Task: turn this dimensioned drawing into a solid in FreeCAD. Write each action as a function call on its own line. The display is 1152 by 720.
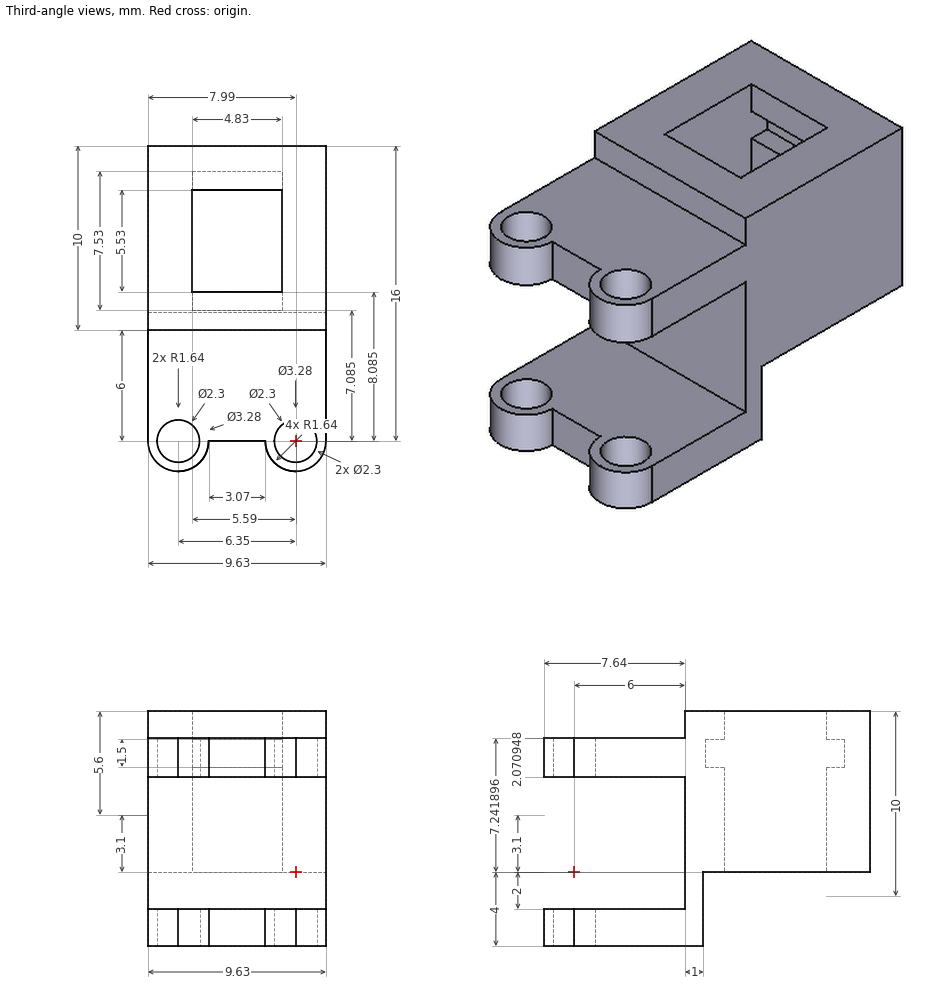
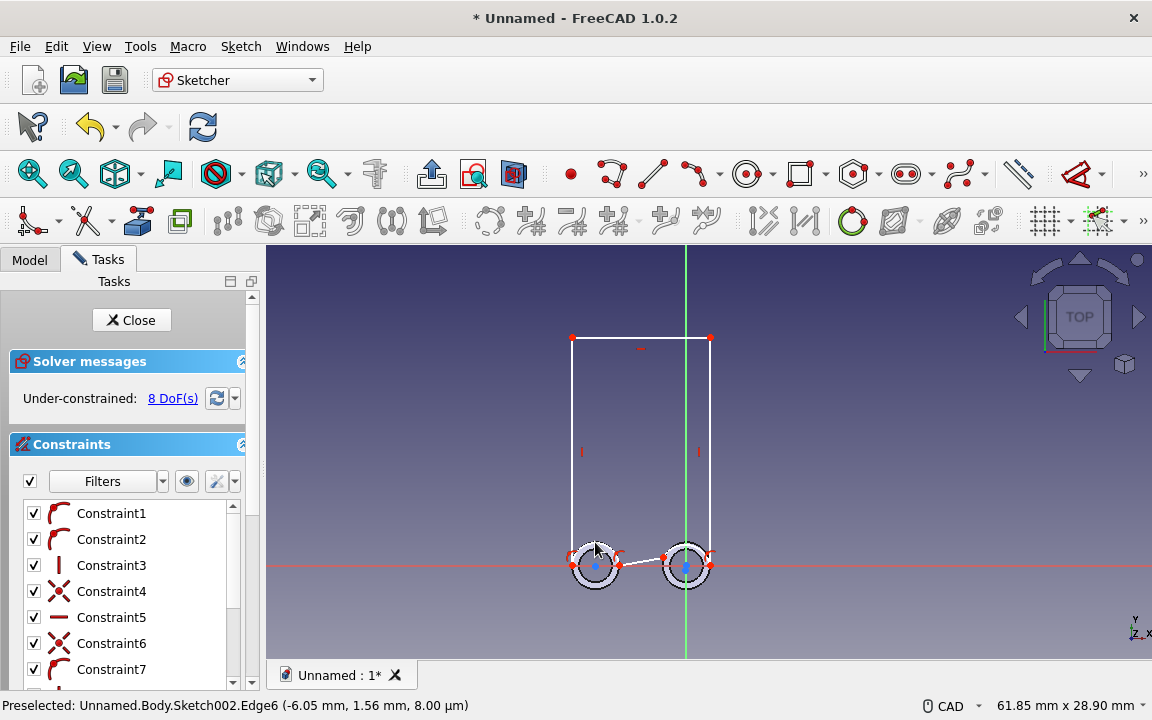
click(710, 497)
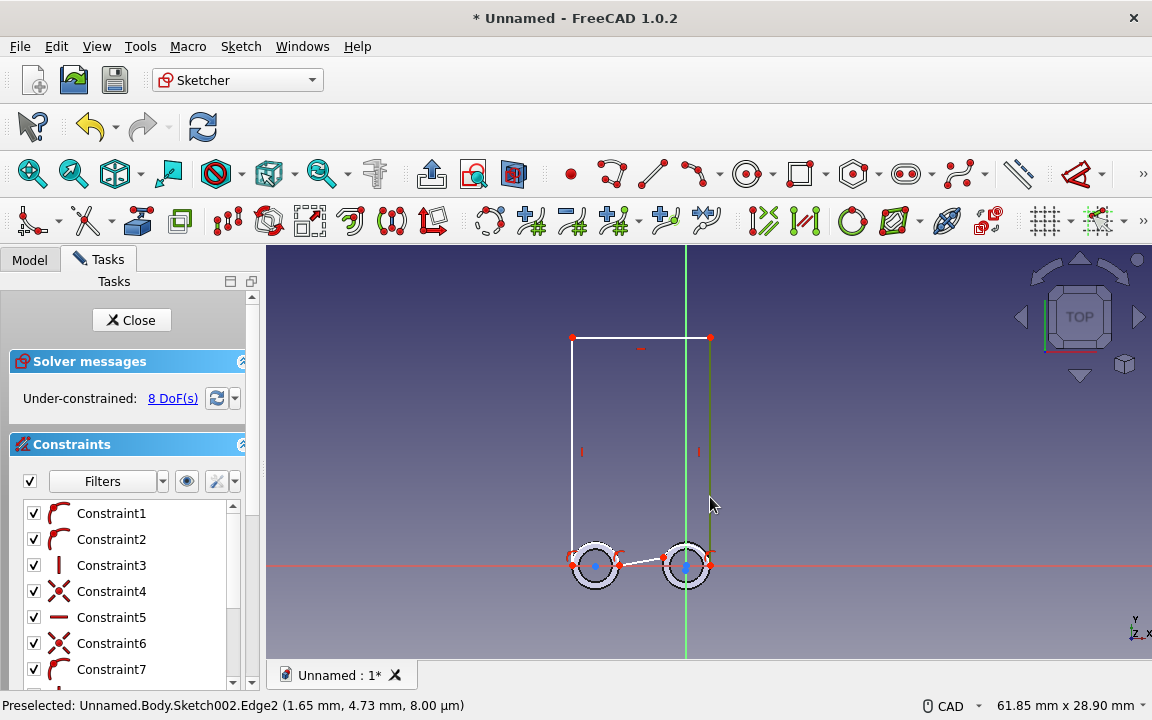
scroll(701, 550, up, 2)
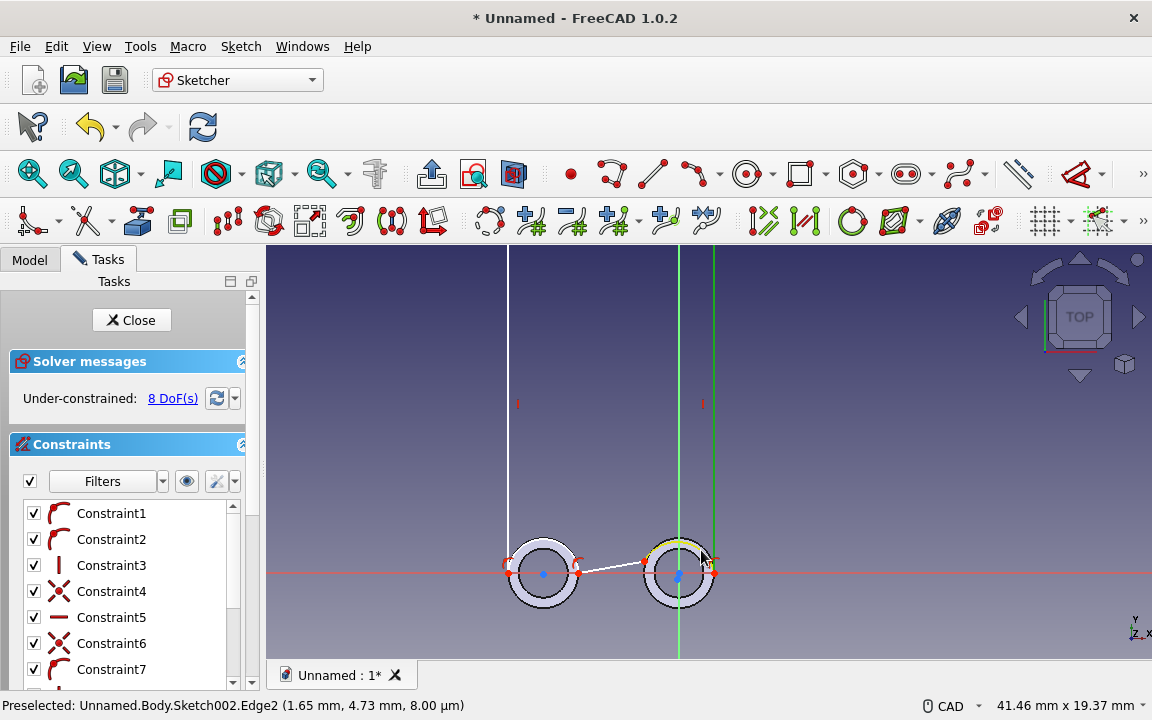
click(700, 550)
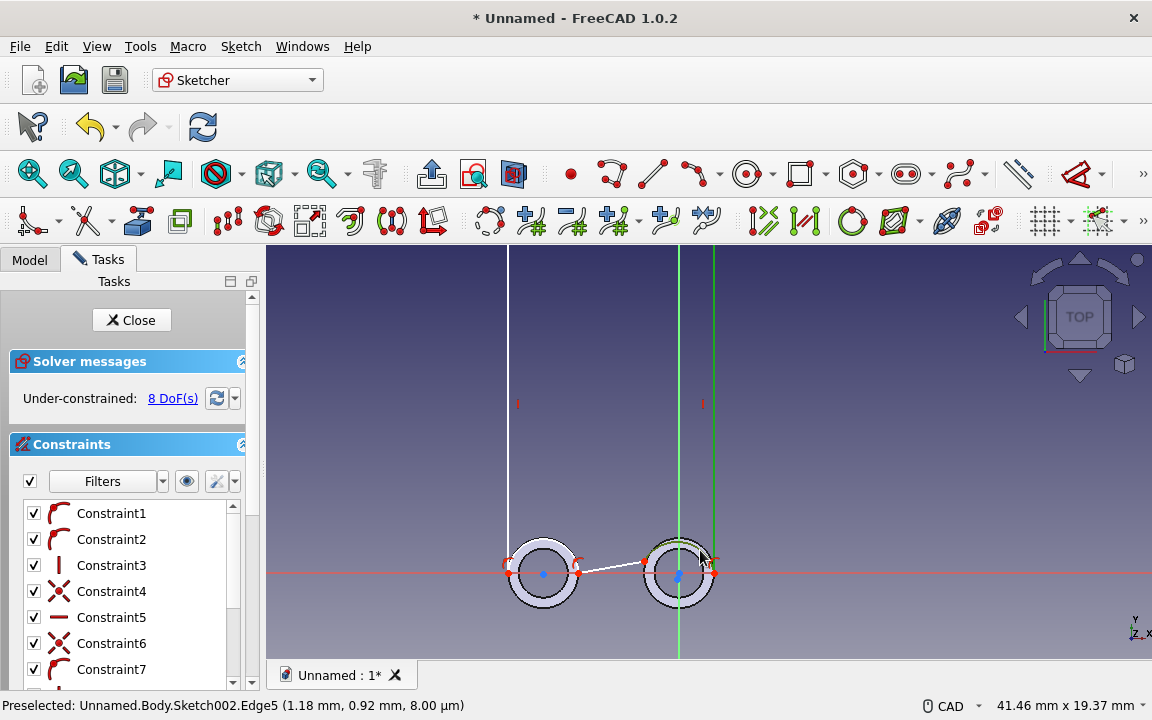
key(t)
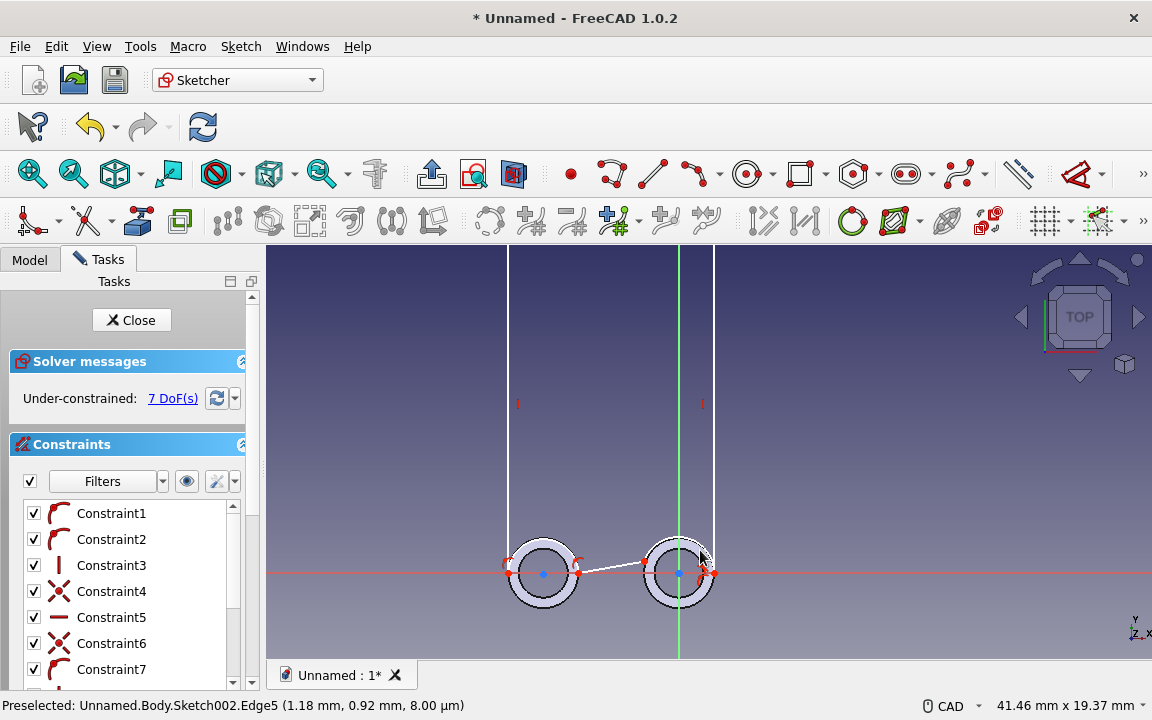
click(508, 335)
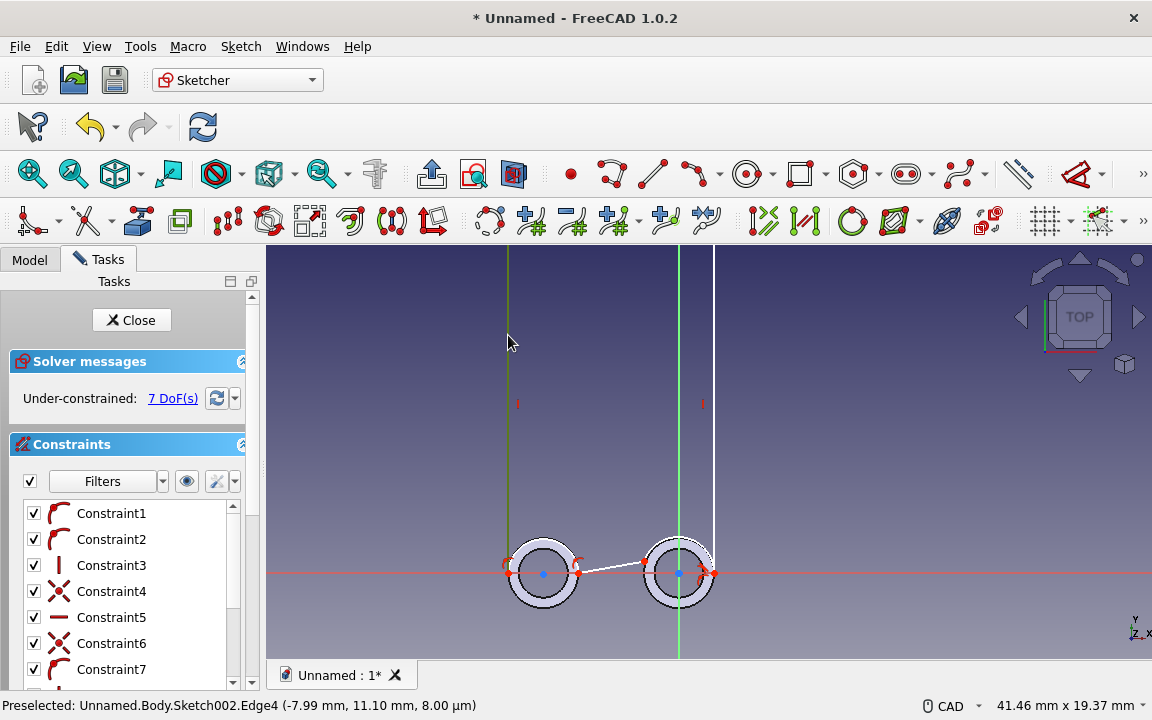
click(564, 546)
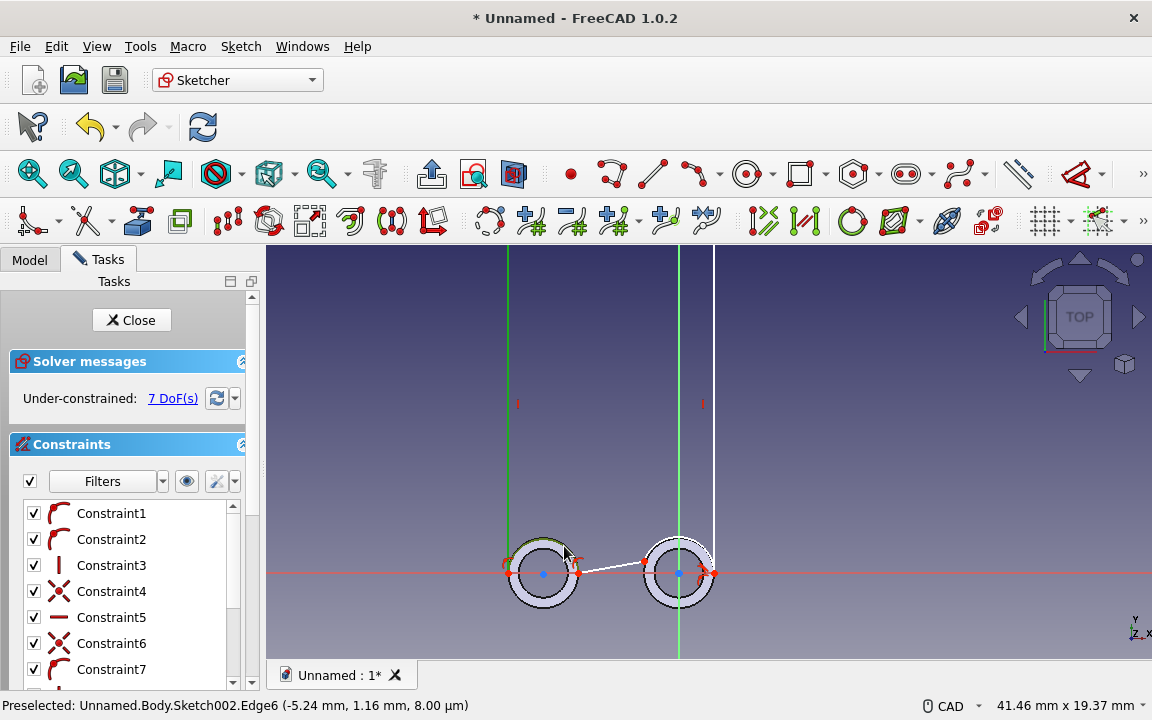
key(t)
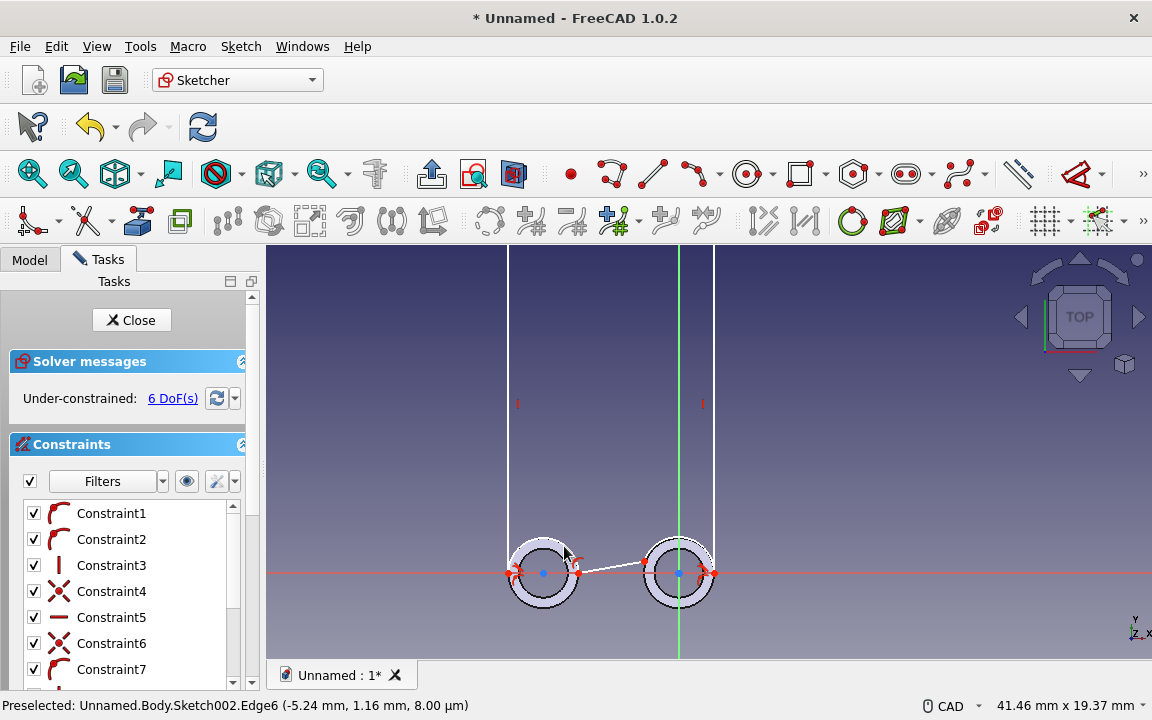
click(598, 570)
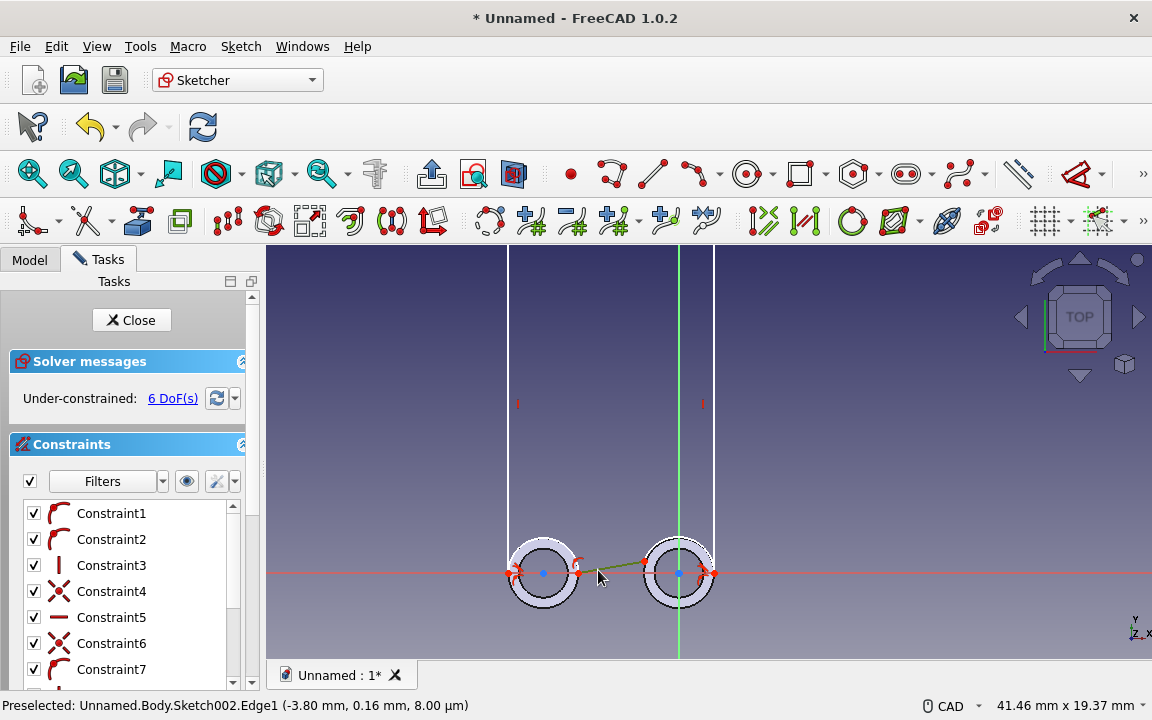
key(h)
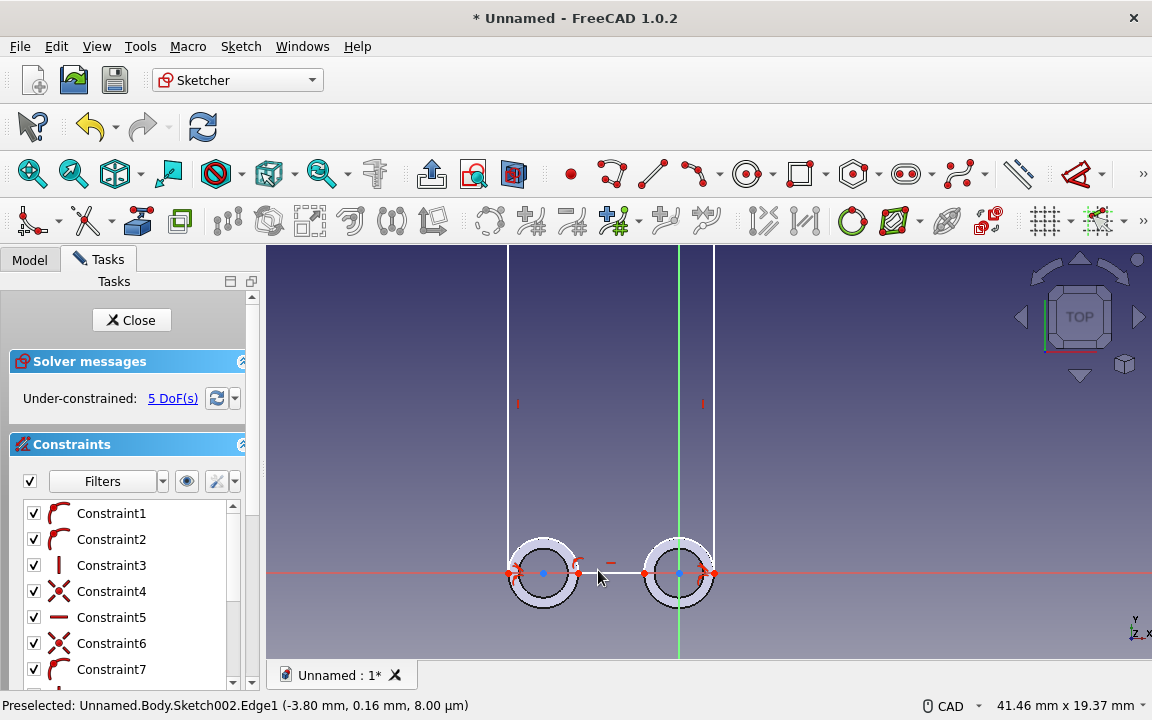
click(700, 545)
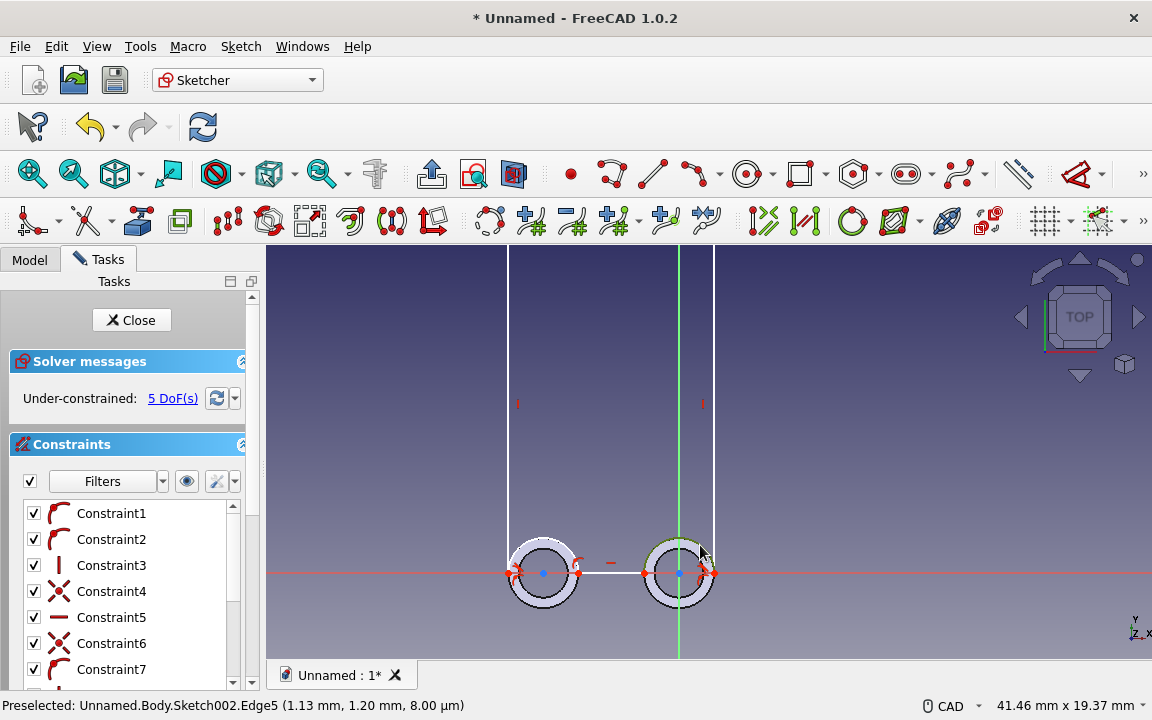
click(564, 545)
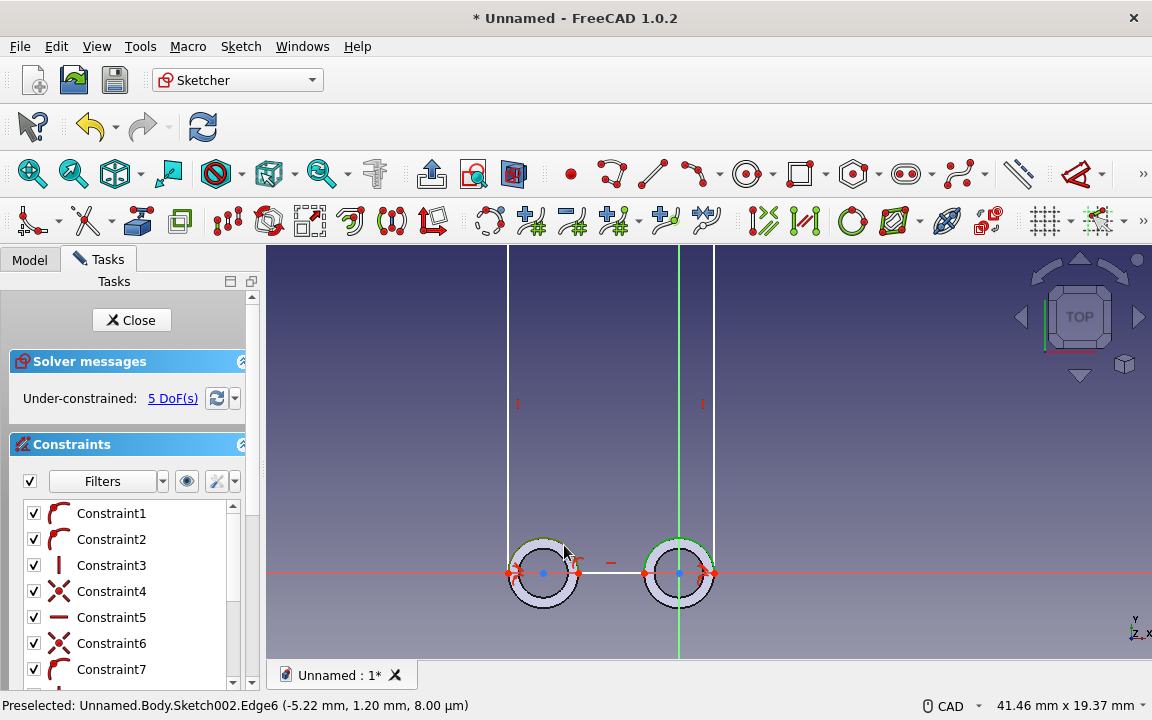
key(e)